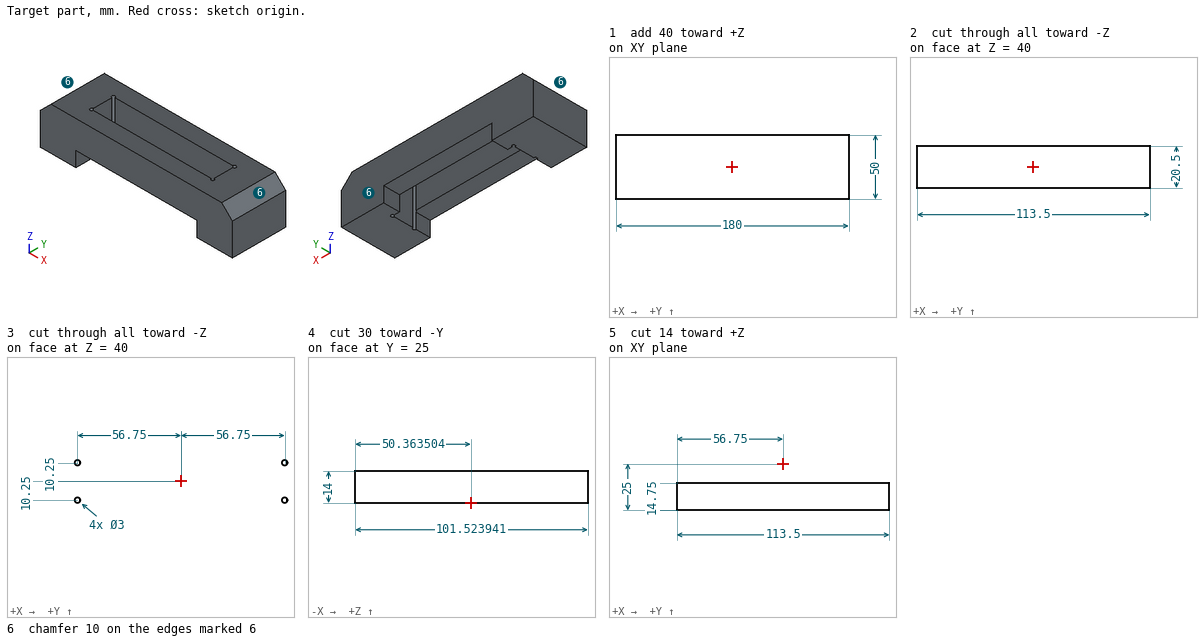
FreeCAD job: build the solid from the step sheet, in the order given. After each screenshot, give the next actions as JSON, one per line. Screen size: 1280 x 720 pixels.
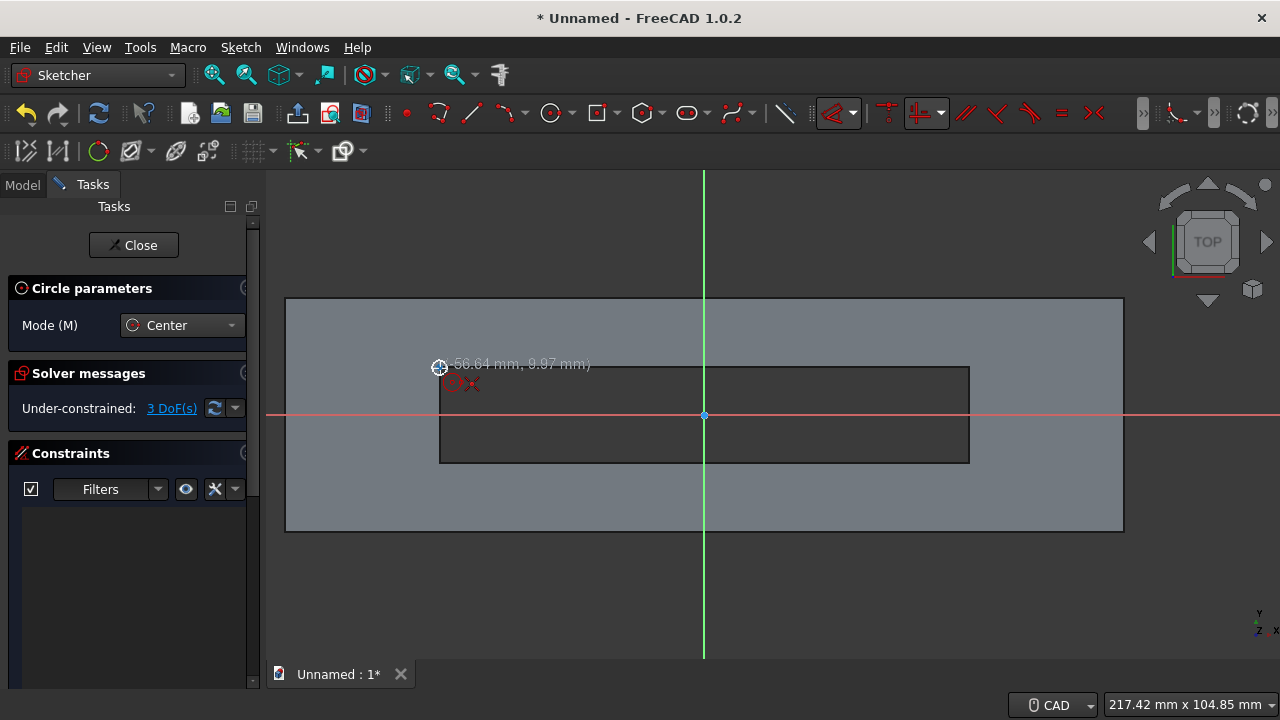
{"action": "scroll", "coordinate": [440, 463], "scroll_direction": "up", "scroll_amount": 6}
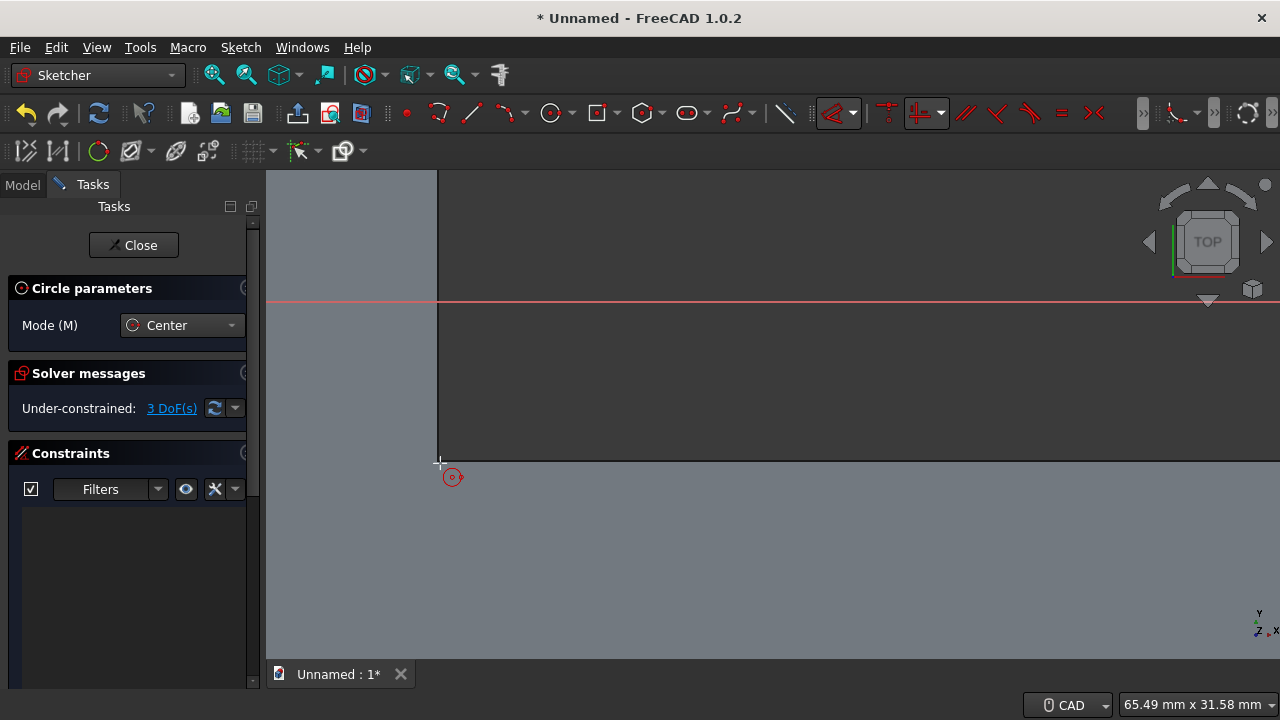
{"action": "left_click", "coordinate": [438, 461]}
{"action": "left_click", "coordinate": [455, 445]}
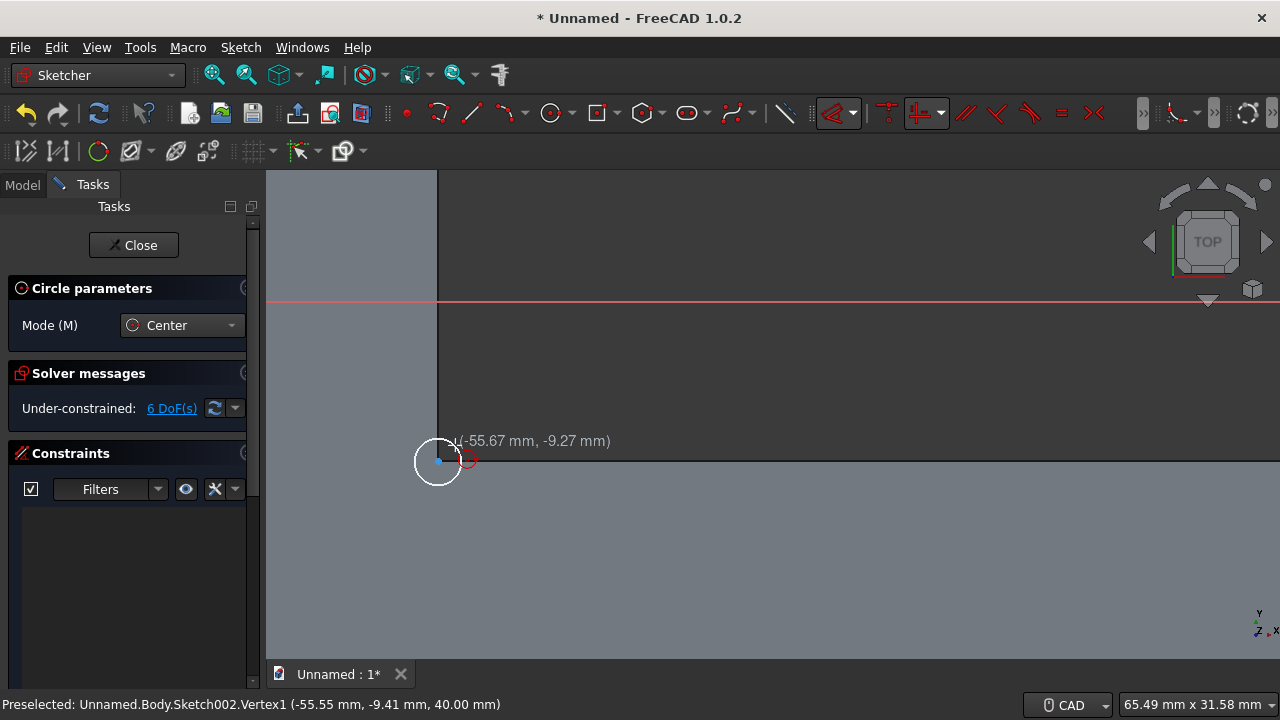
{"action": "scroll", "coordinate": [440, 463], "scroll_direction": "down", "scroll_amount": 6}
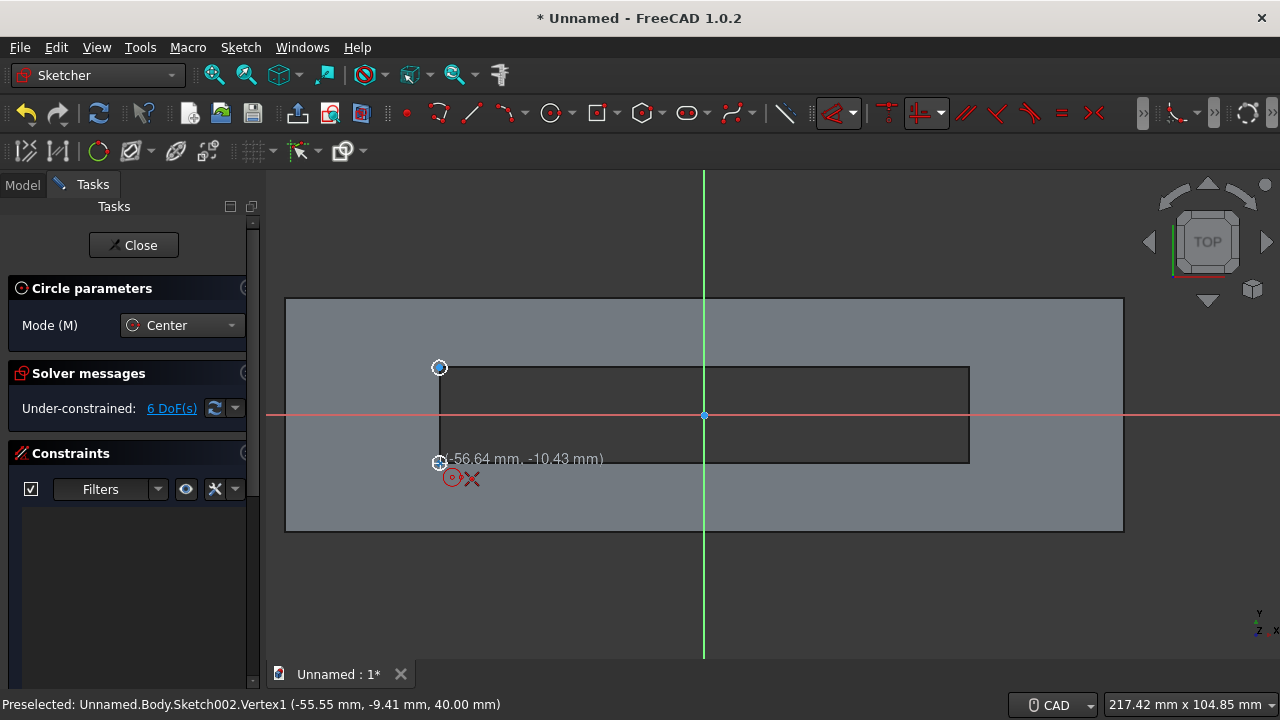
{"action": "scroll", "coordinate": [969, 367], "scroll_direction": "up", "scroll_amount": 6}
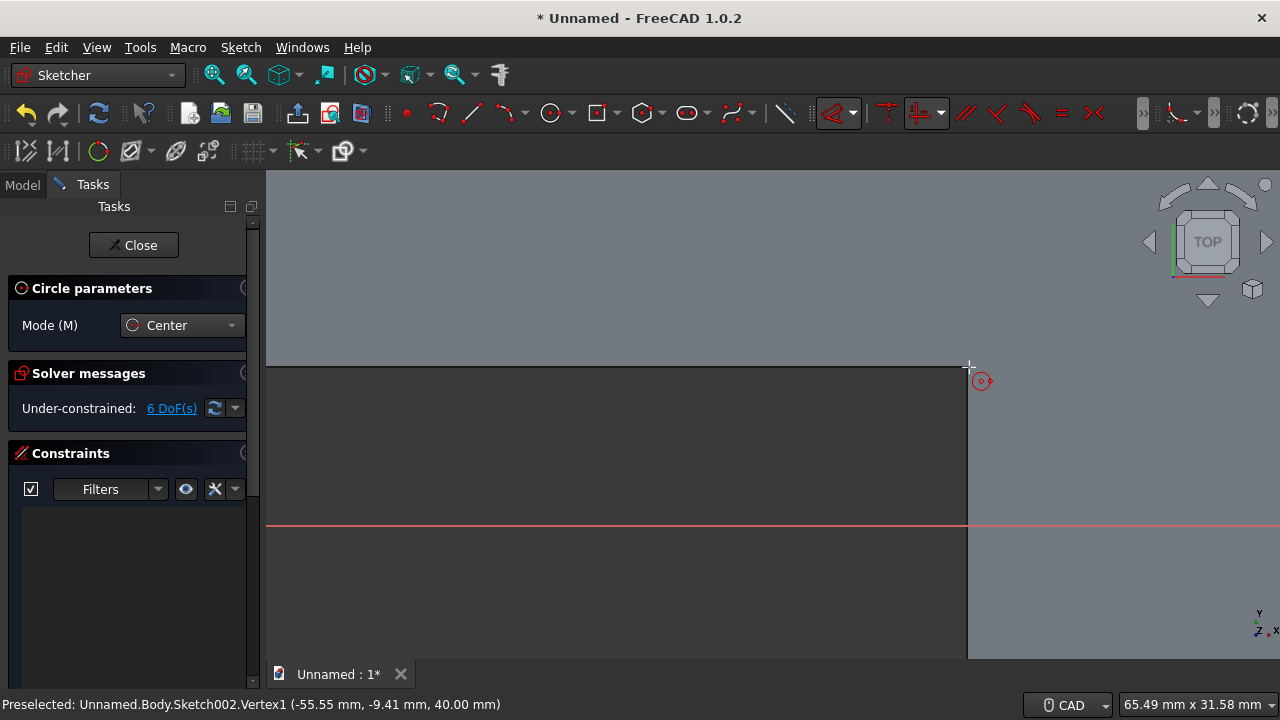
{"action": "left_click", "coordinate": [967, 367]}
{"action": "left_click", "coordinate": [984, 351]}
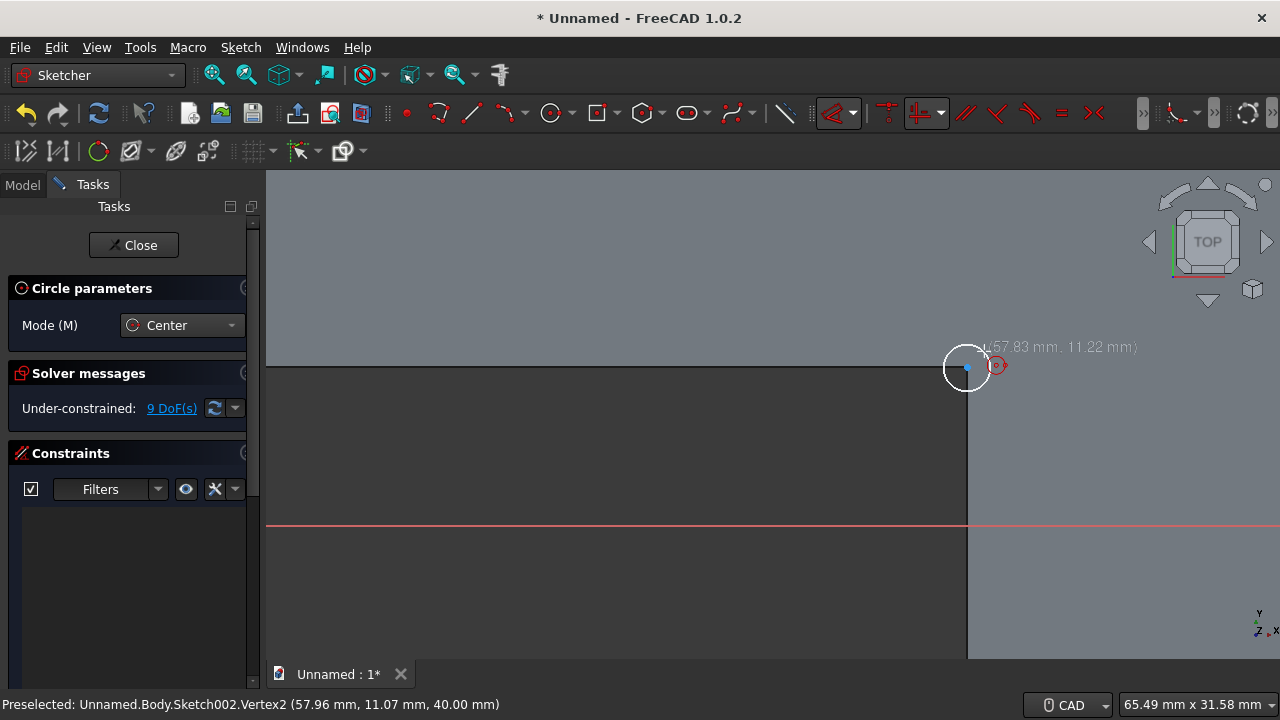
{"action": "scroll", "coordinate": [970, 367], "scroll_direction": "down", "scroll_amount": 6}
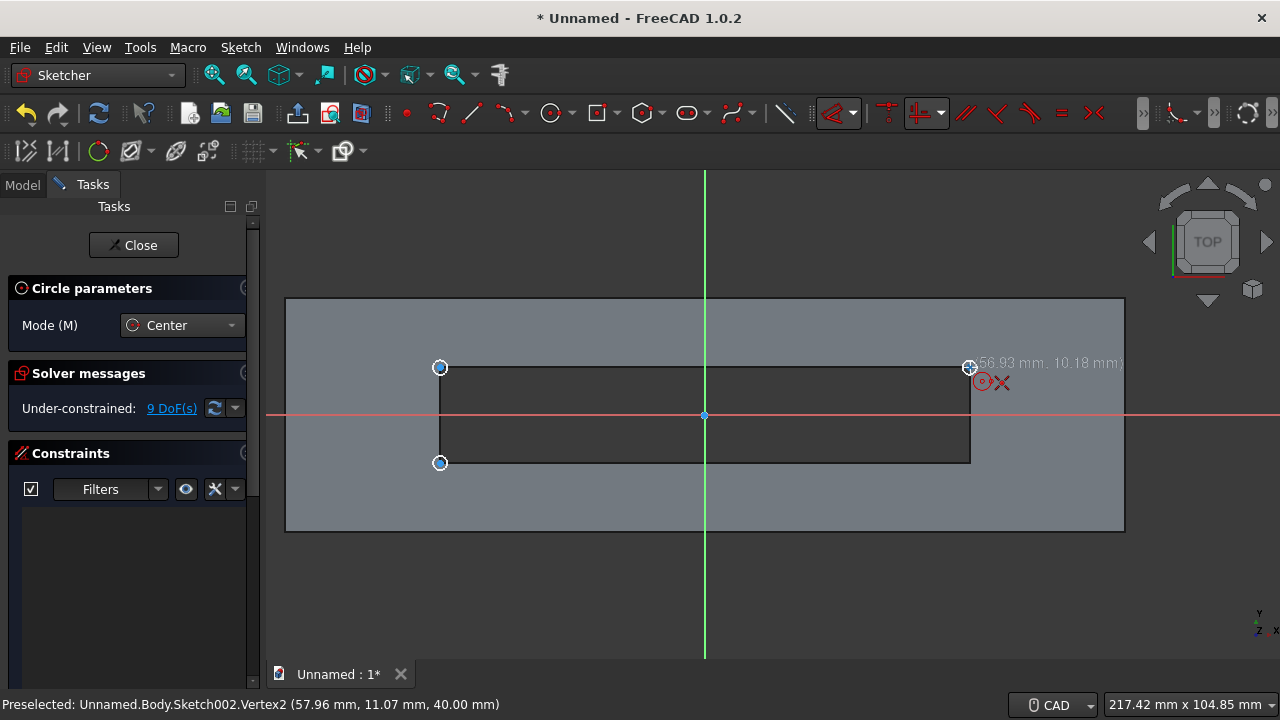
{"action": "scroll", "coordinate": [970, 463], "scroll_direction": "up", "scroll_amount": 6}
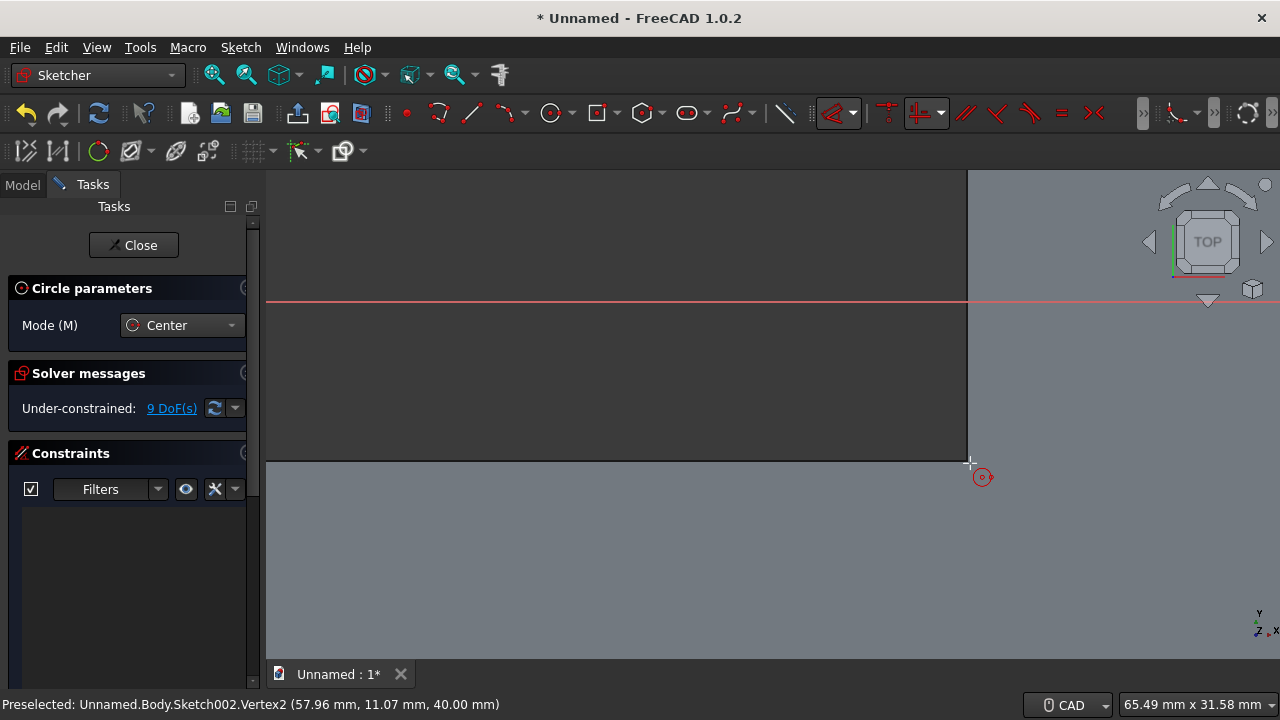
{"action": "left_click", "coordinate": [967, 461]}
{"action": "left_click", "coordinate": [984, 445]}
{"action": "key", "text": "Escape"}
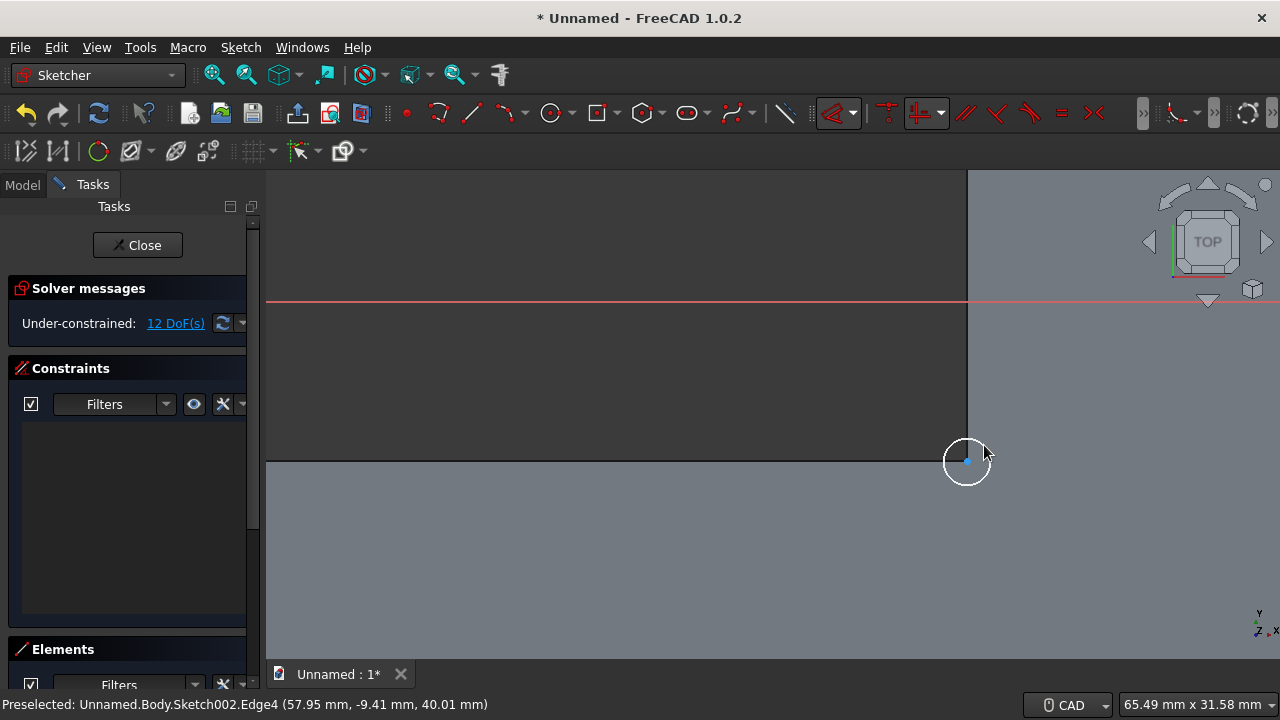
{"action": "scroll", "coordinate": [970, 463], "scroll_direction": "down", "scroll_amount": 6}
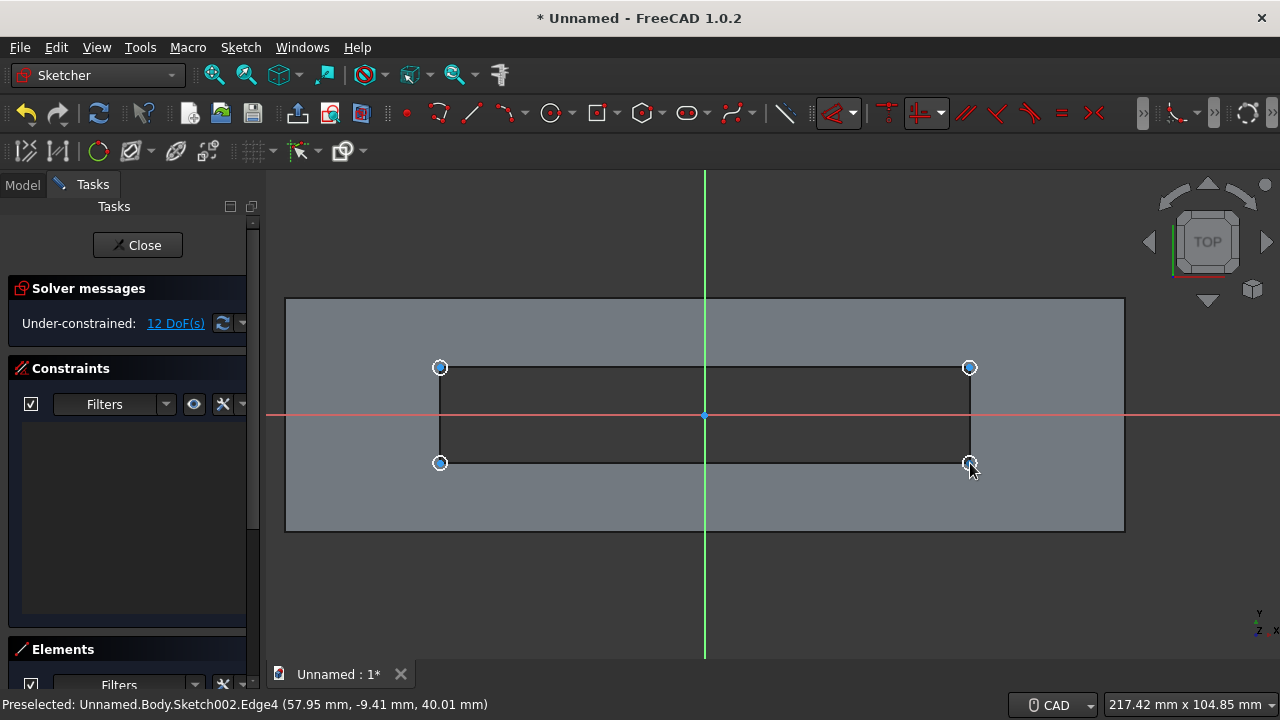
{"action": "scroll", "coordinate": [445, 363], "scroll_direction": "up", "scroll_amount": 4}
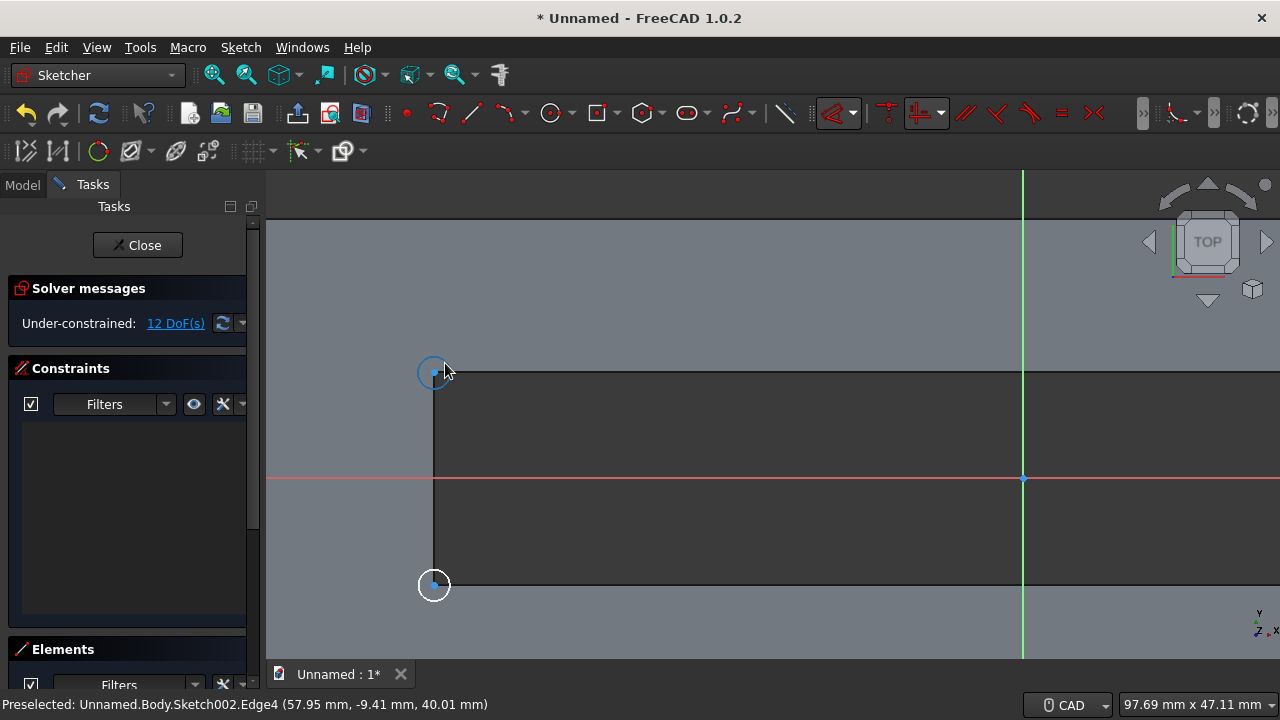
{"action": "left_click", "coordinate": [445, 362]}